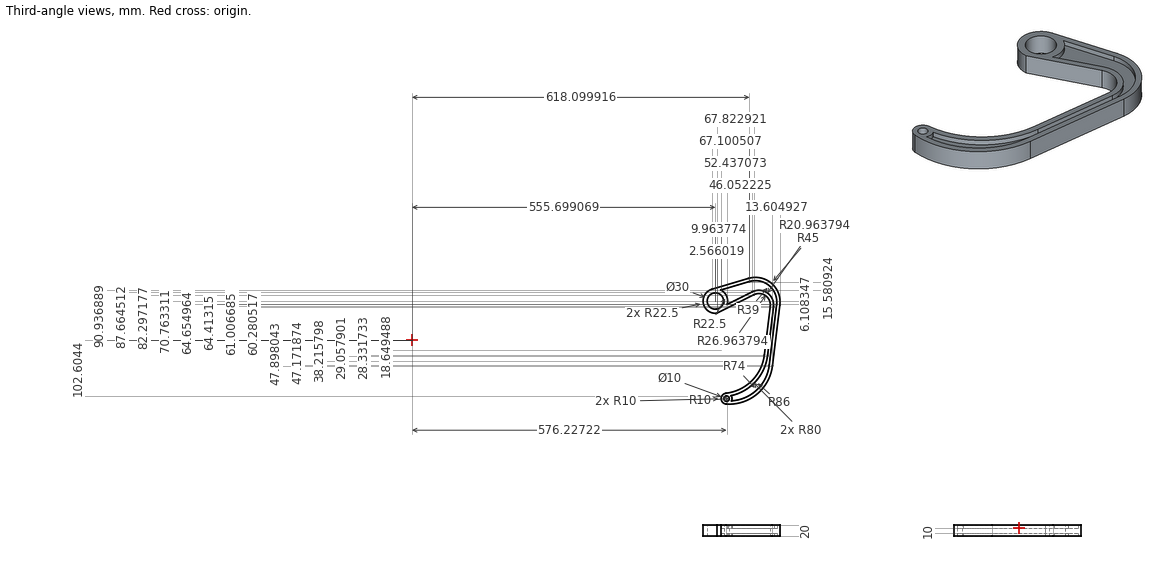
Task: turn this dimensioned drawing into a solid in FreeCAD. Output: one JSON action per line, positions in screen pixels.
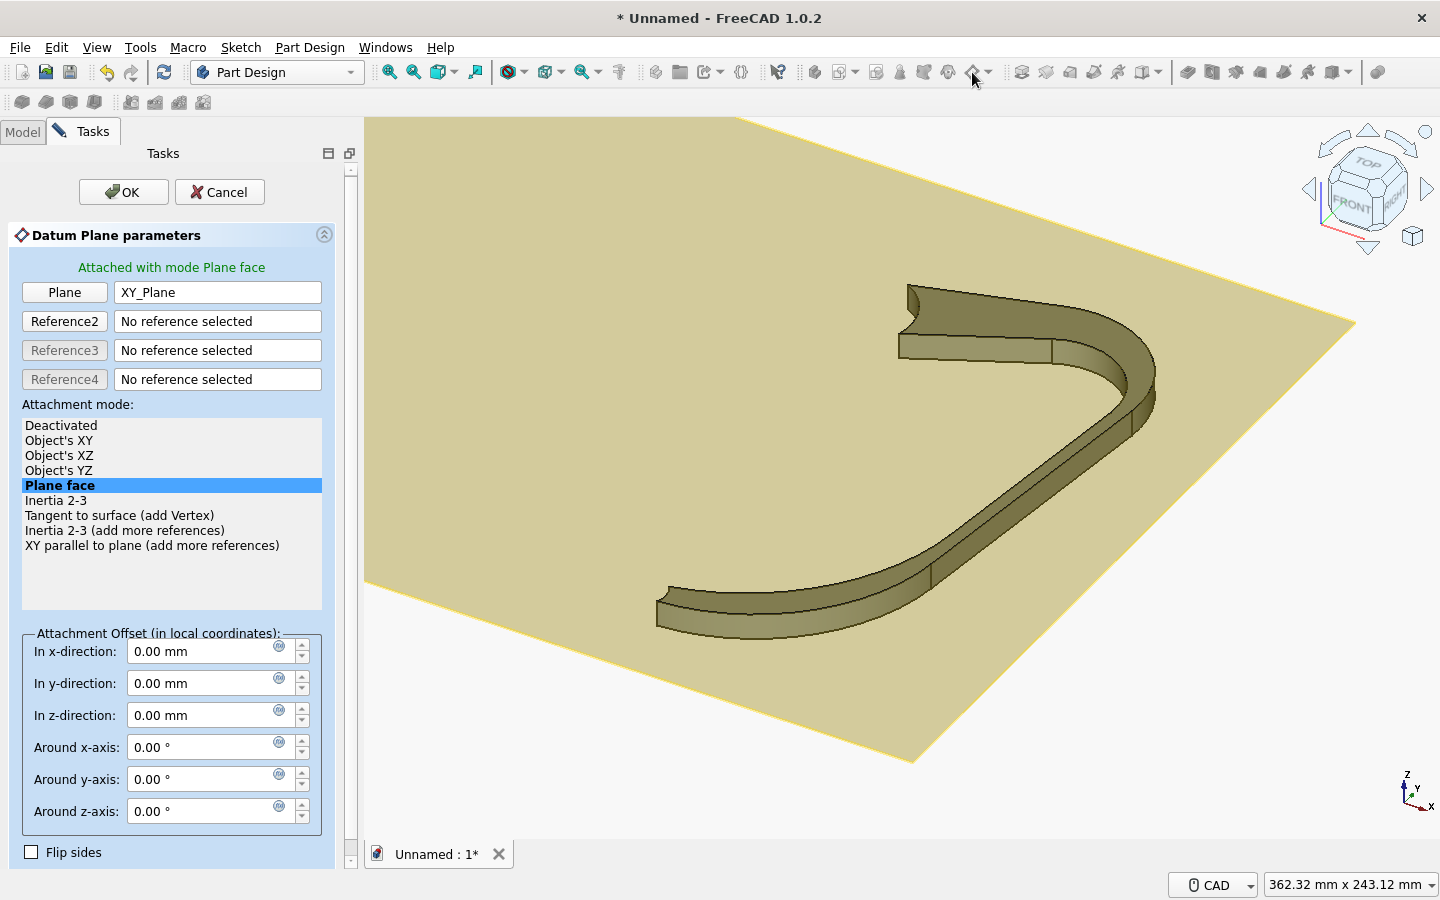
{"action": "triple_click", "coordinate": [210, 715]}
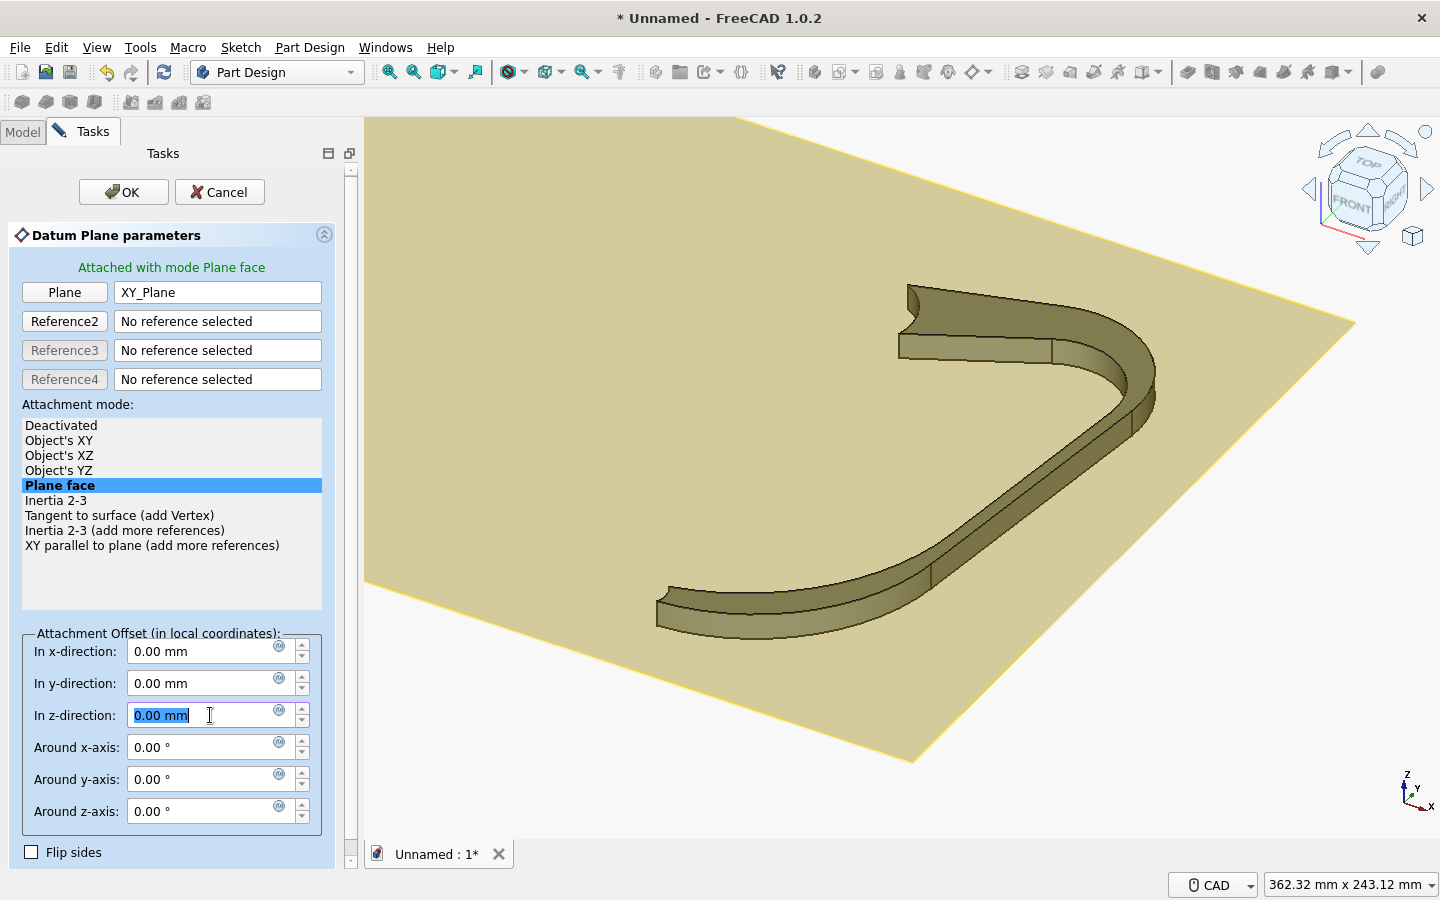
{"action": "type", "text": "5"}
{"action": "key", "text": "Tab"}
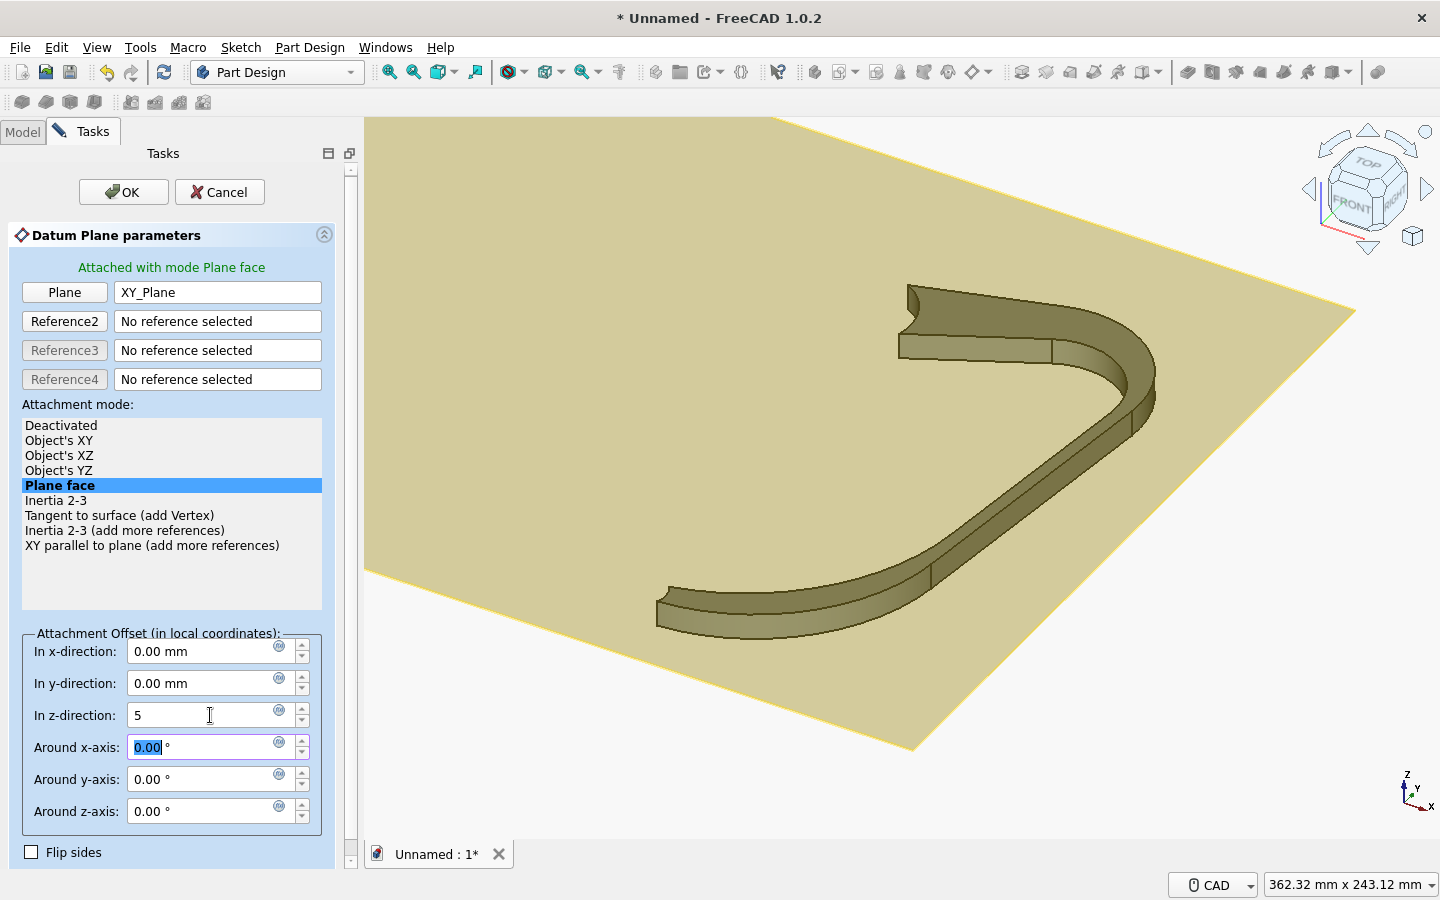
{"action": "left_click", "coordinate": [124, 192]}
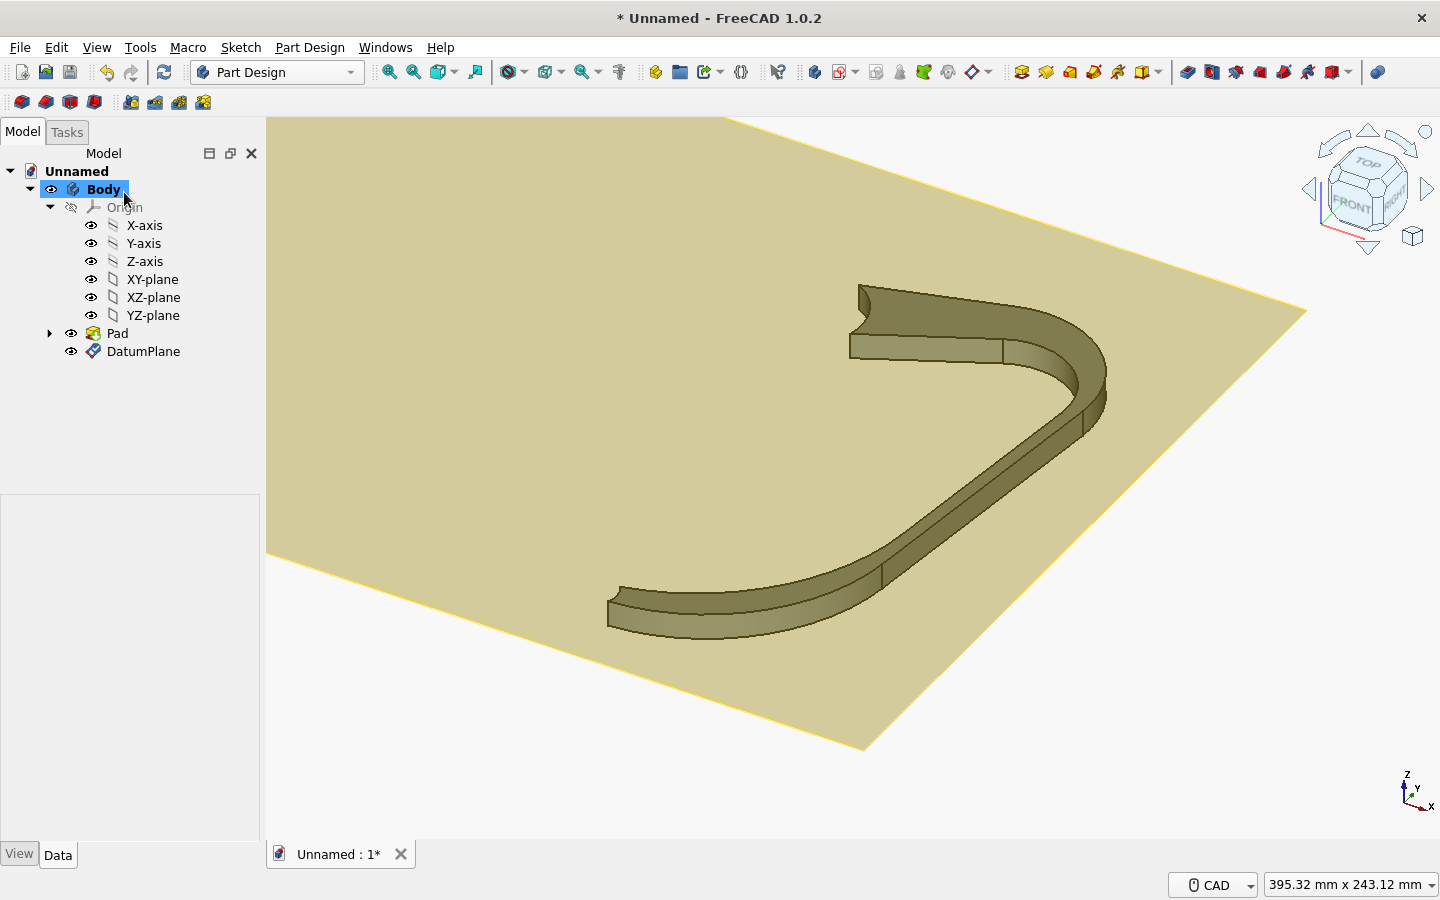
{"action": "left_click", "coordinate": [116, 351]}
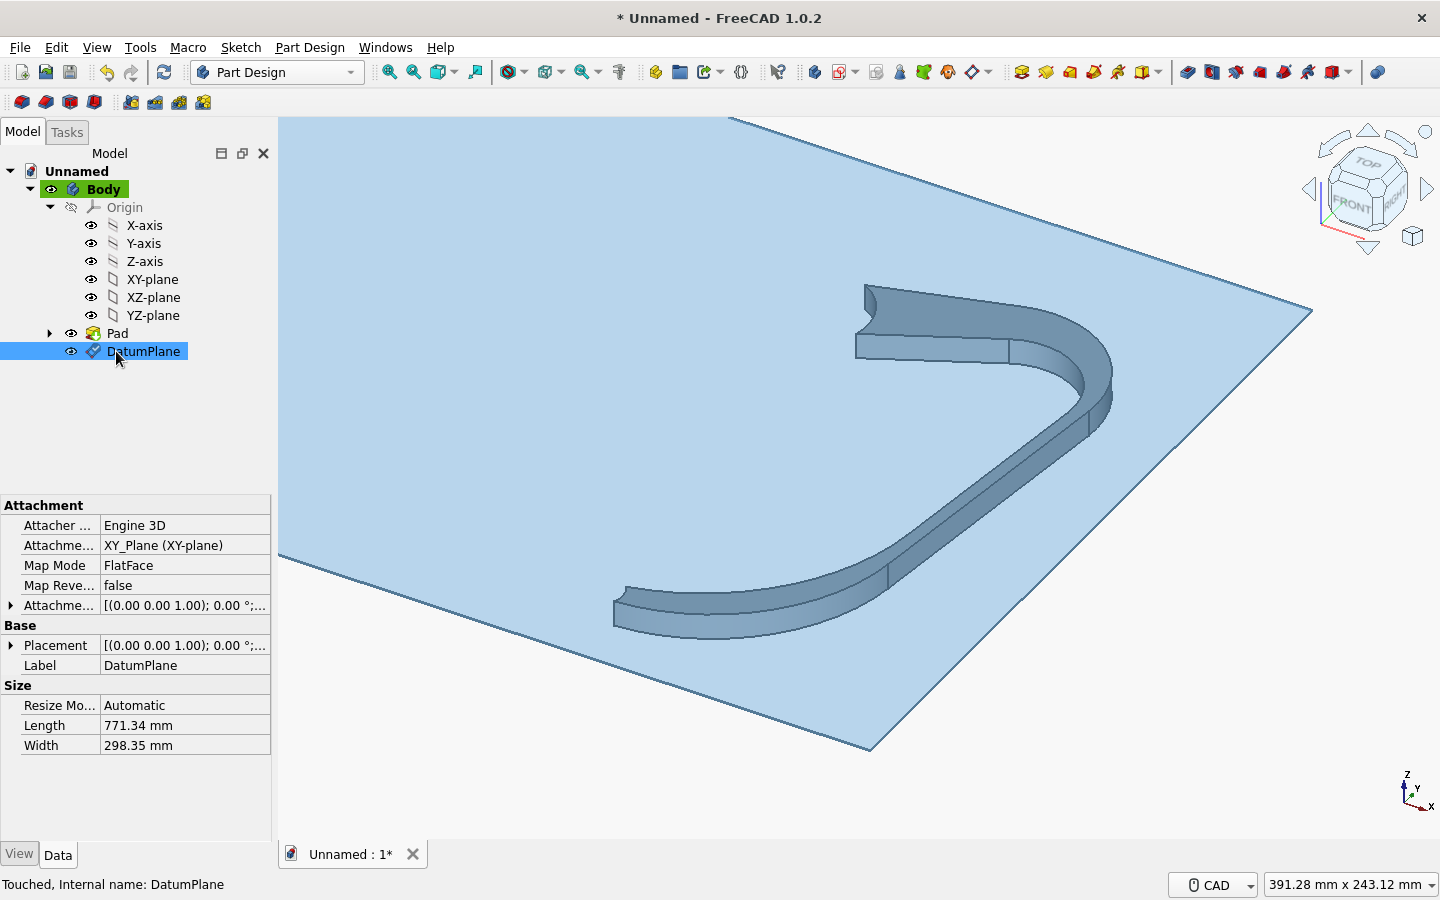
{"action": "left_click", "coordinate": [840, 72]}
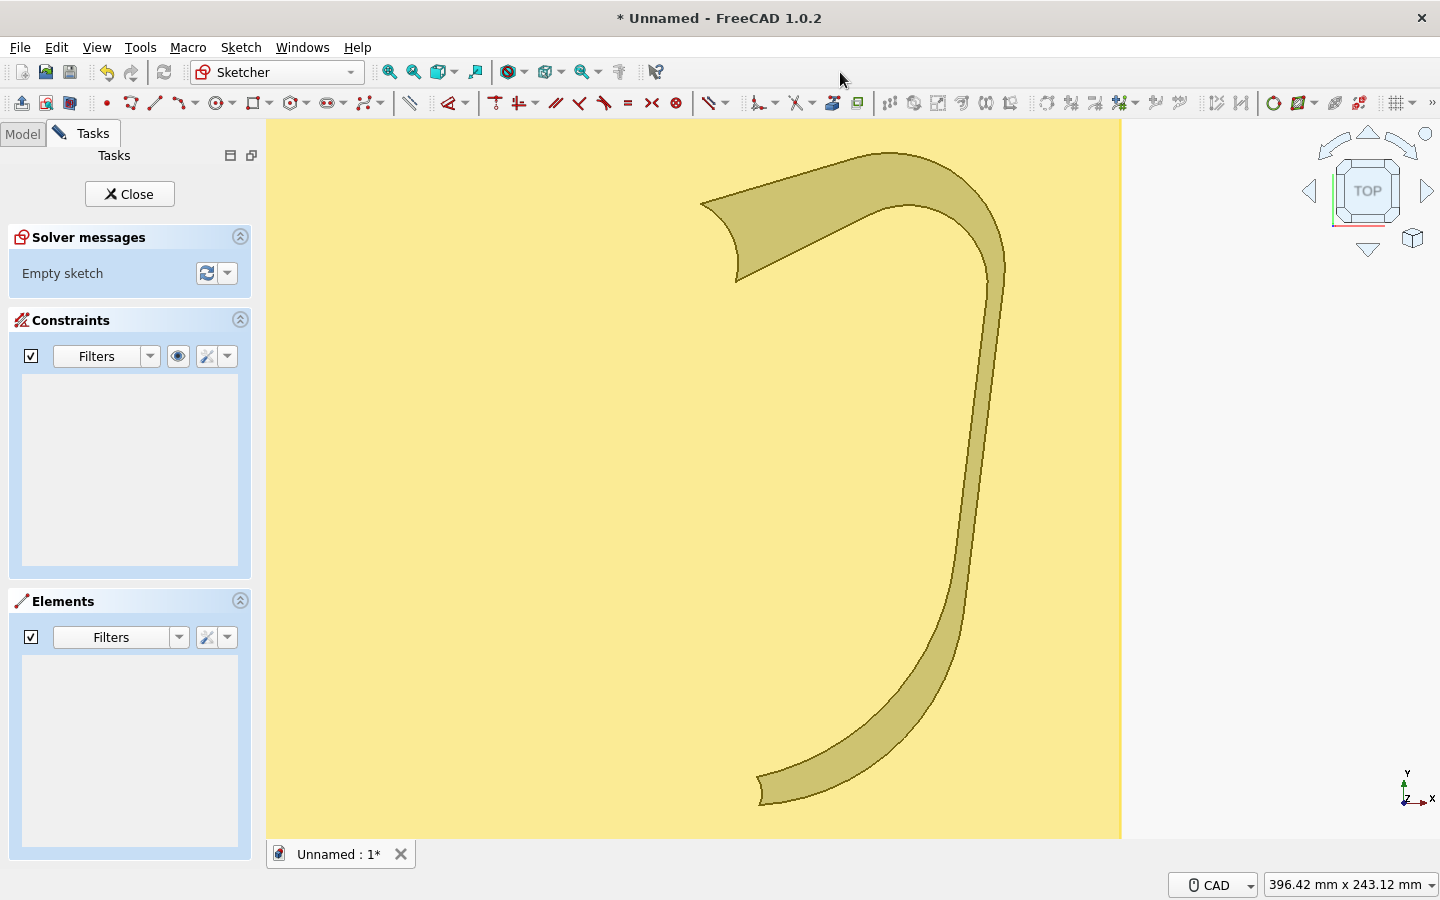
{"action": "scroll", "coordinate": [724, 474], "scroll_direction": "down", "scroll_amount": 2}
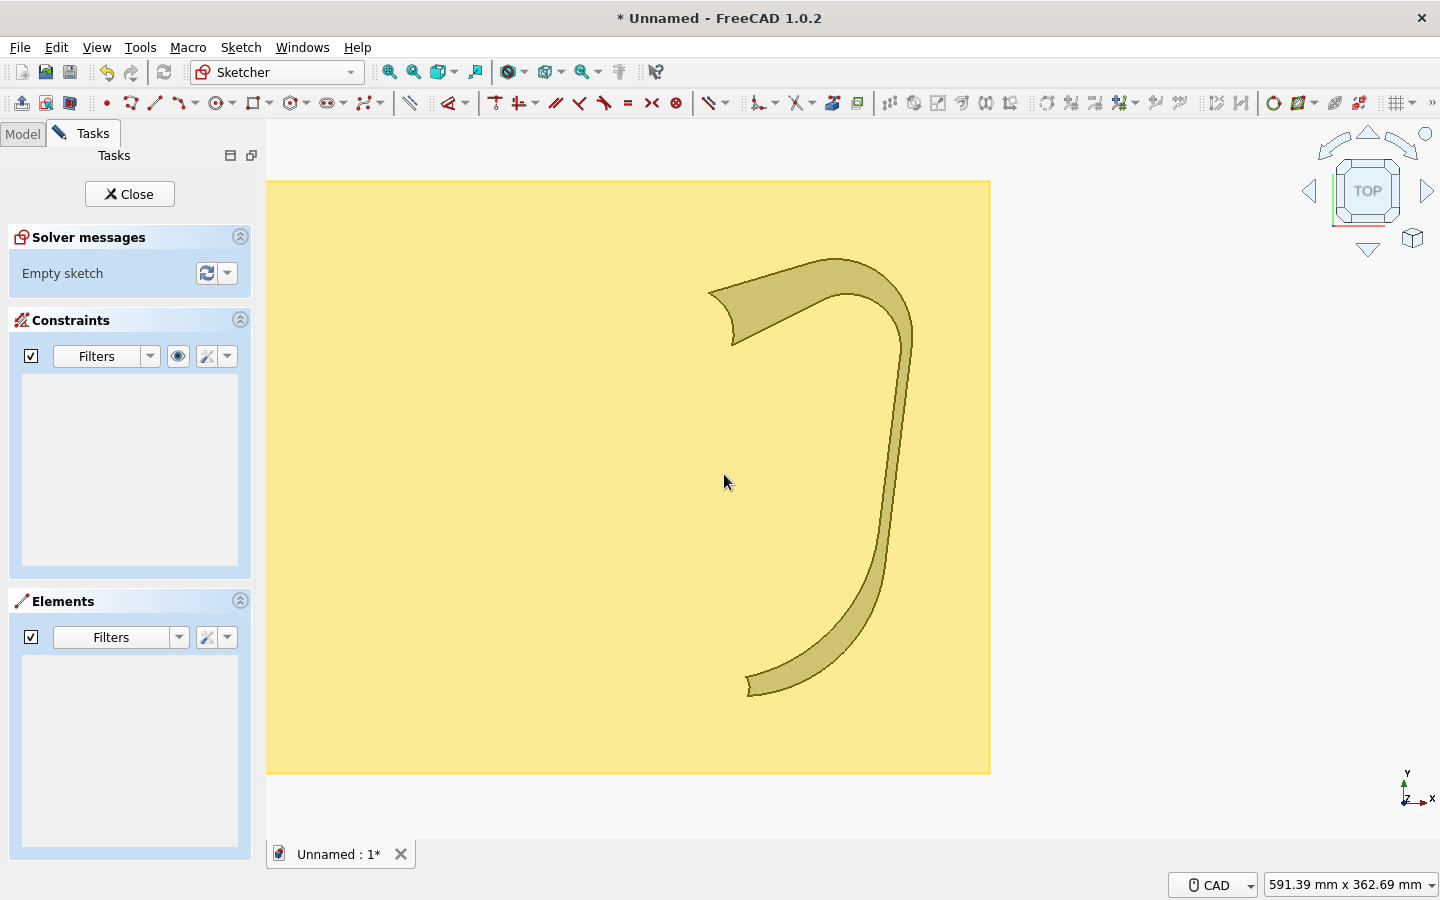
{"action": "left_click", "coordinate": [156, 104]}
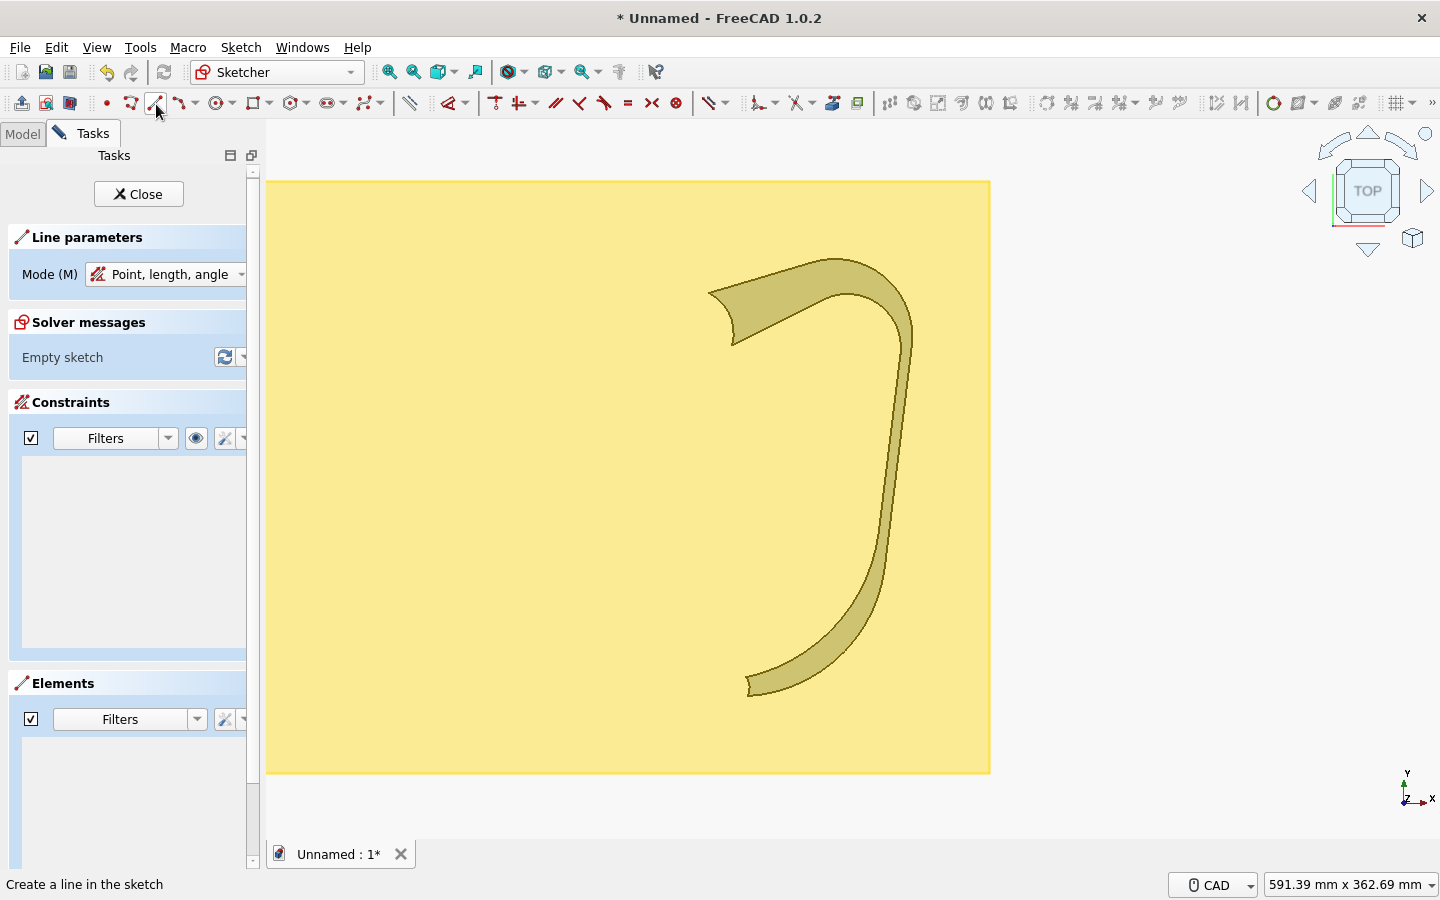
{"action": "left_click", "coordinate": [810, 251]}
{"action": "left_click", "coordinate": [676, 290]}